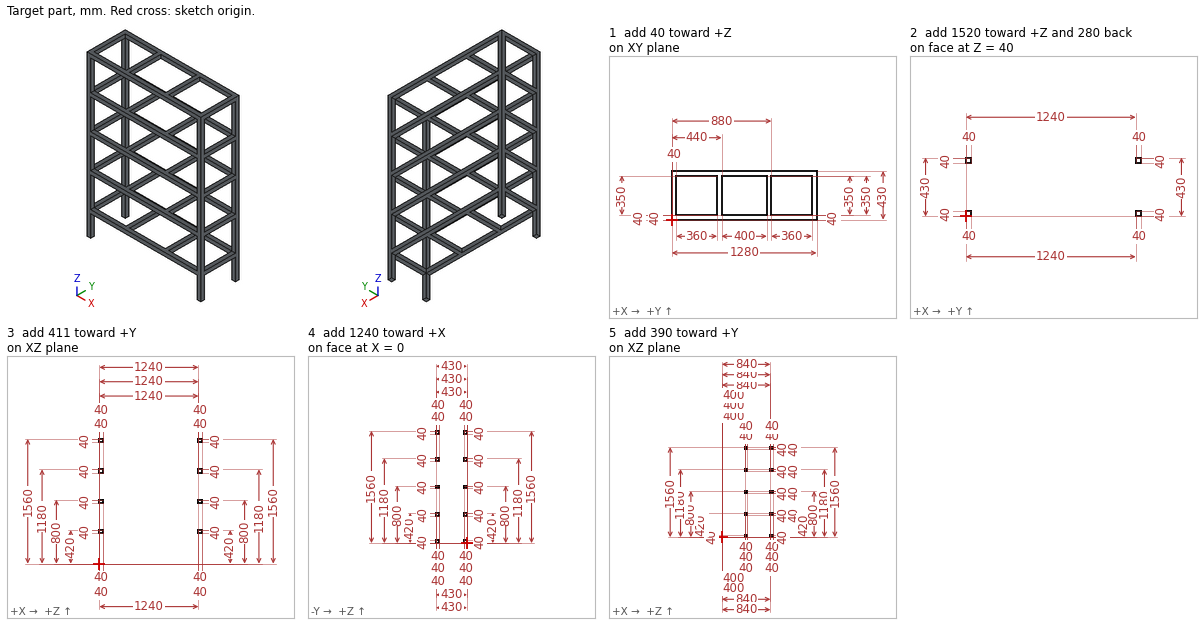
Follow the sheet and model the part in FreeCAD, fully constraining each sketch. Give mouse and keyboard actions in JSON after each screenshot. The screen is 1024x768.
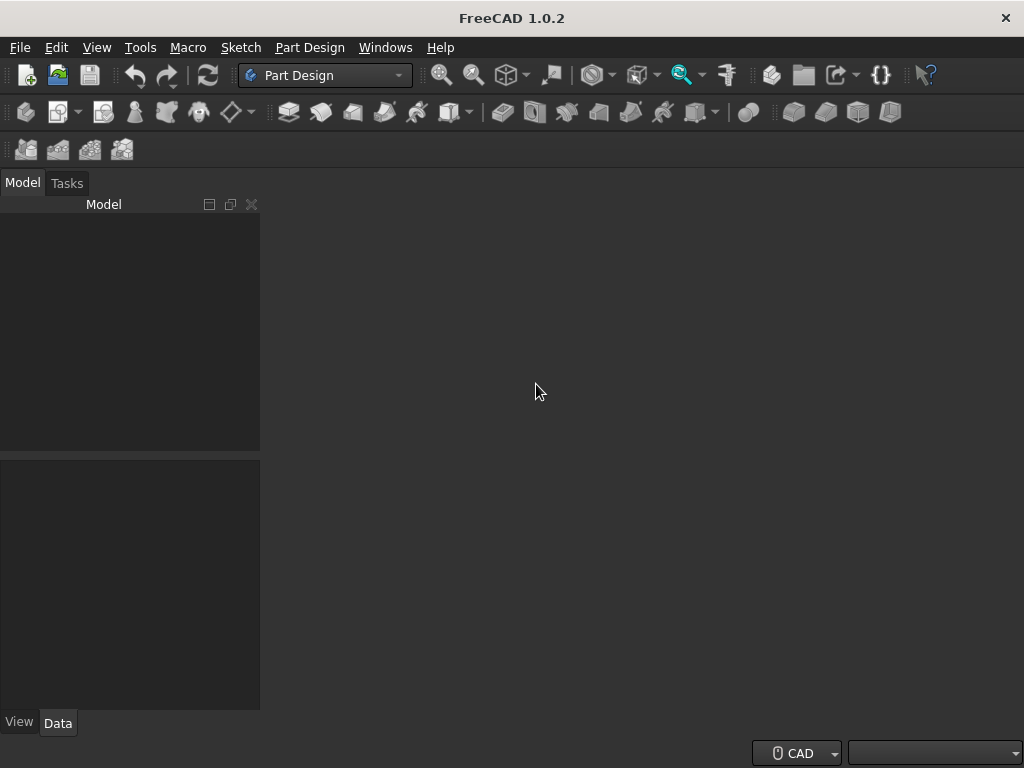
{"action": "left_click", "coordinate": [26, 76]}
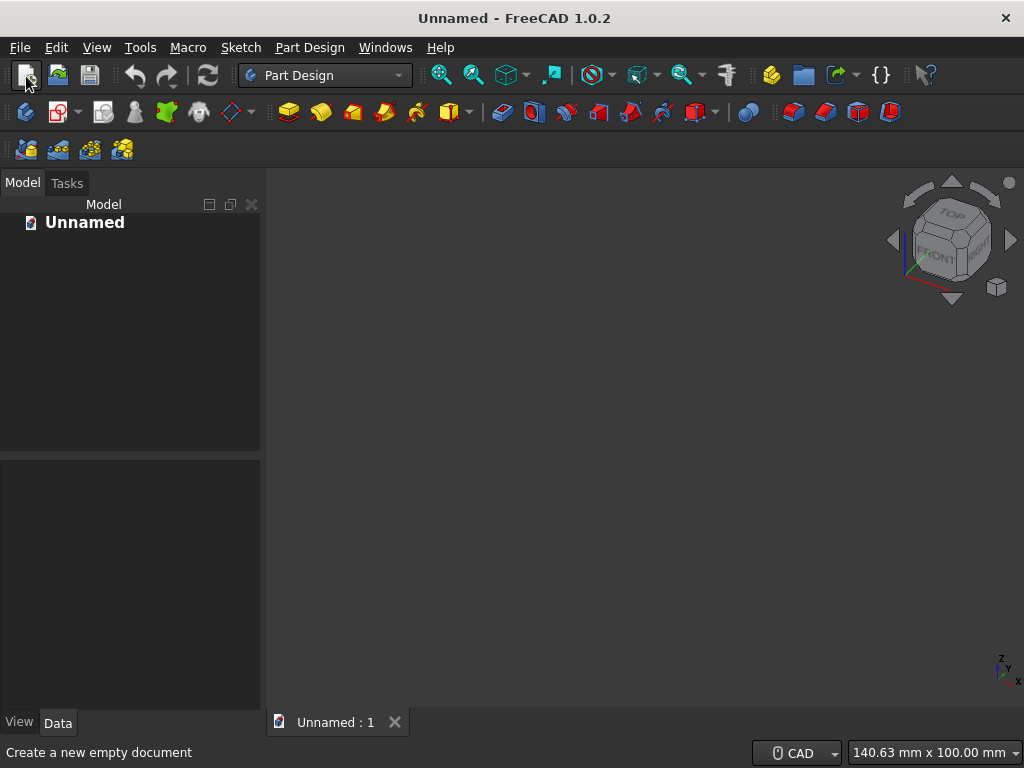
{"action": "left_click", "coordinate": [58, 112]}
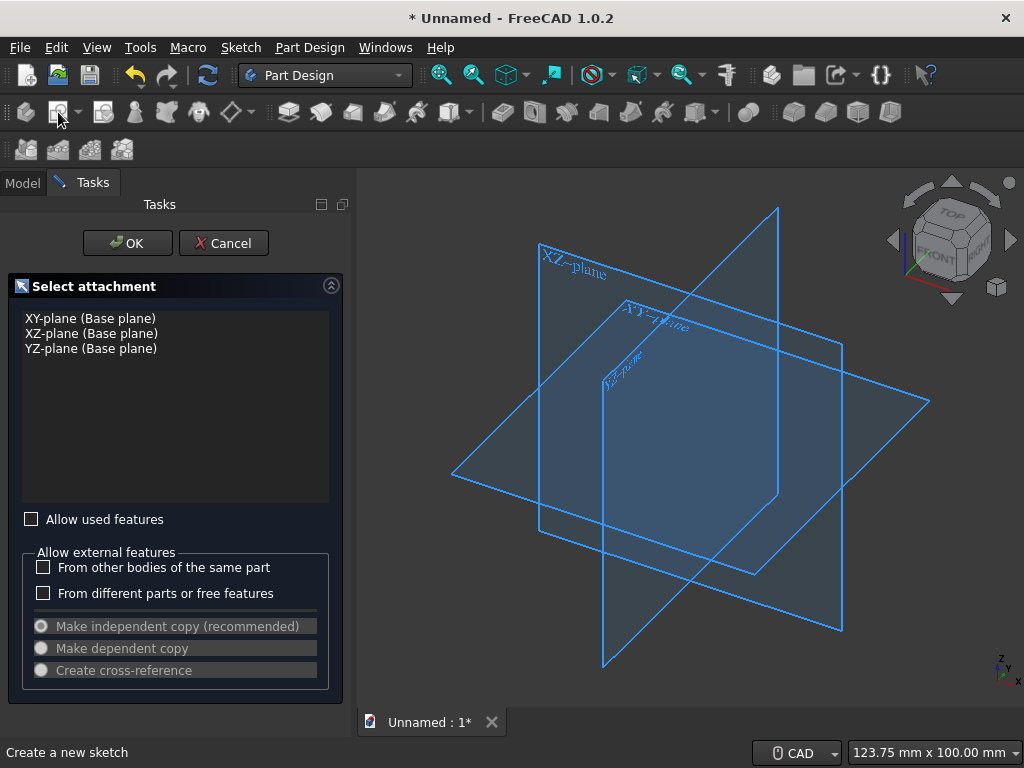
{"action": "left_click", "coordinate": [82, 318]}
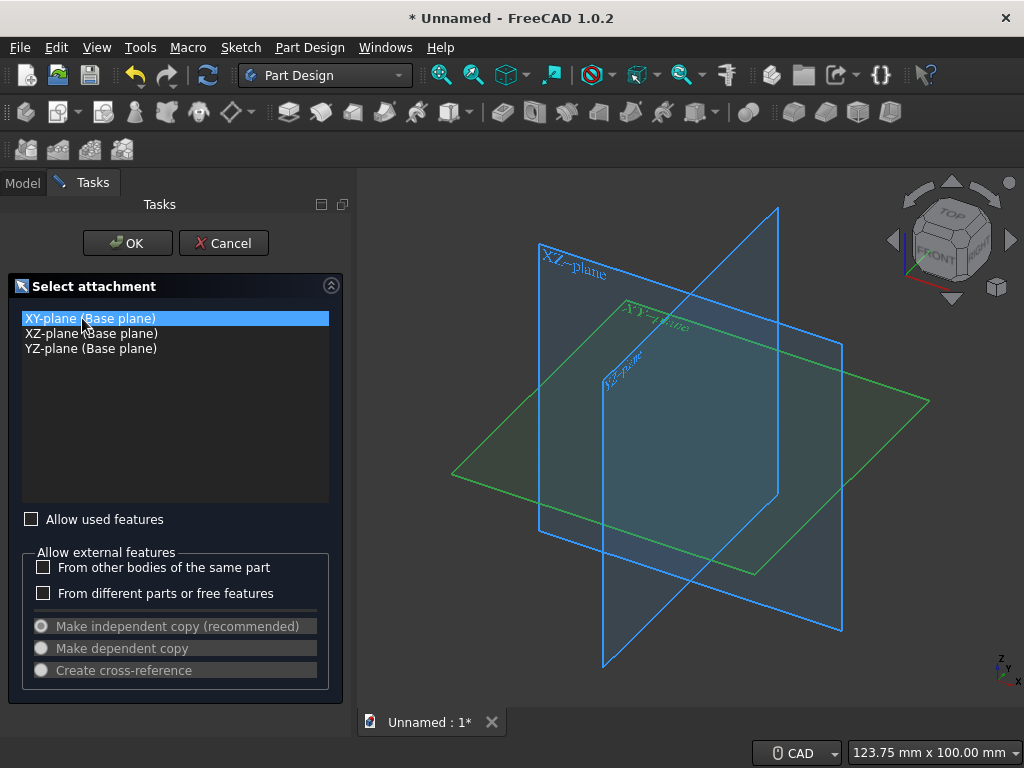
{"action": "left_click", "coordinate": [128, 243]}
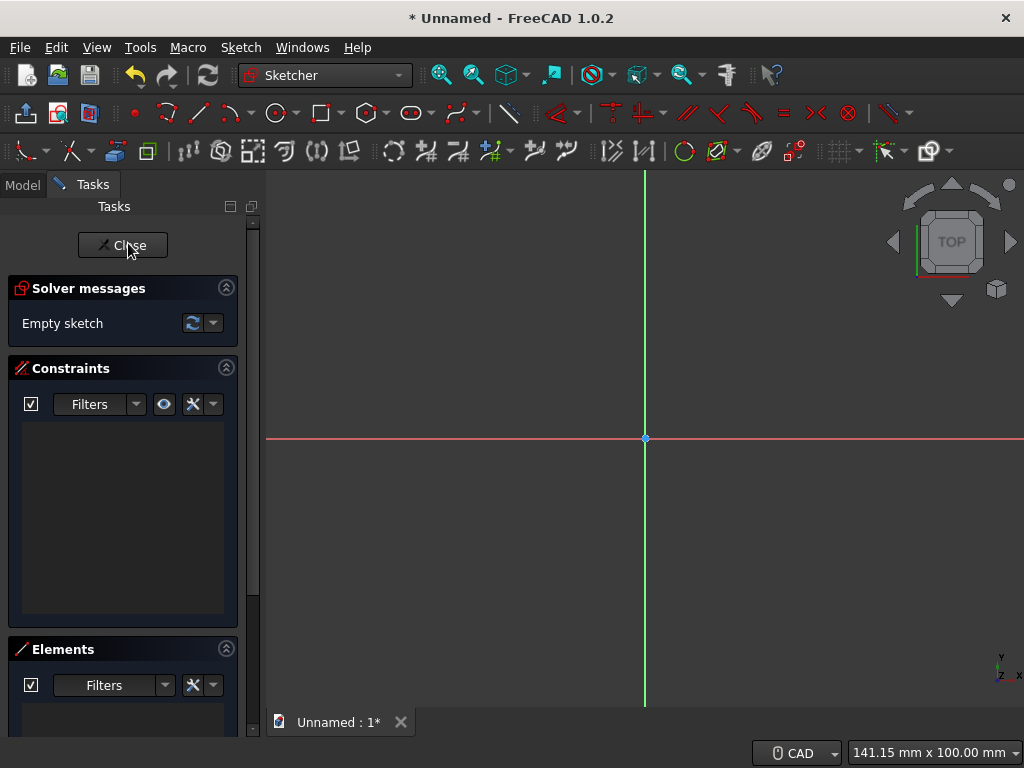
{"action": "scroll", "coordinate": [350, 513], "scroll_direction": "down", "scroll_amount": 14}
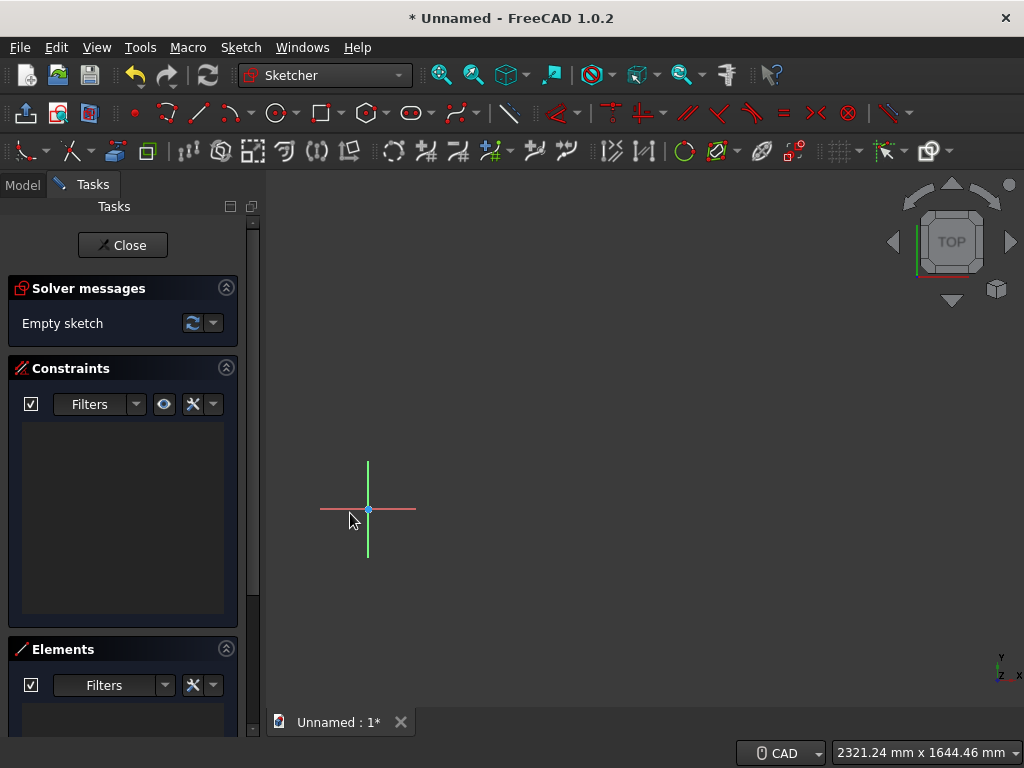
{"action": "left_click", "coordinate": [322, 114]}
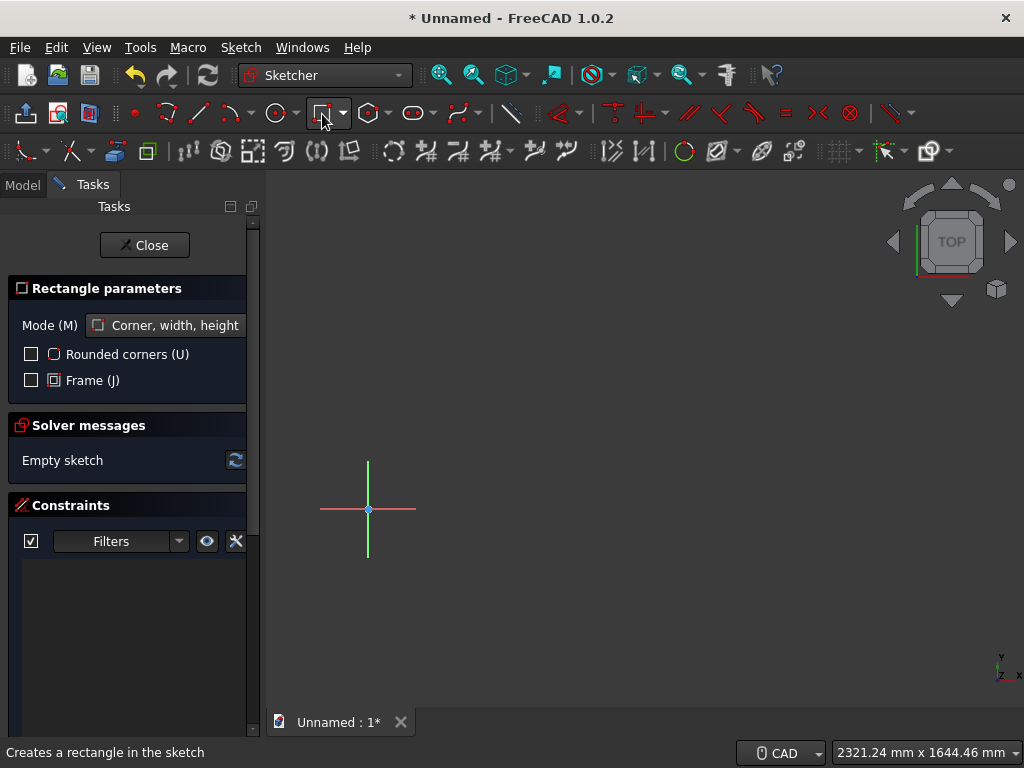
{"action": "left_click", "coordinate": [368, 509]}
{"action": "mouse_move", "coordinate": [786, 369]}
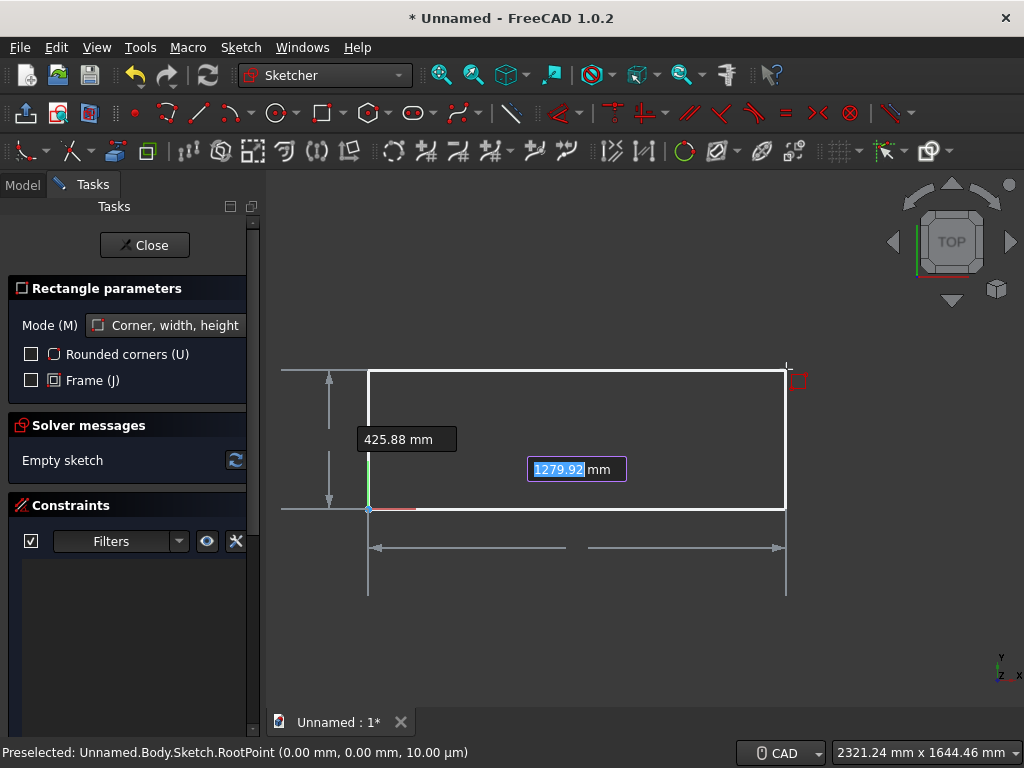
{"action": "type", "text": "1280"}
{"action": "key", "text": "Tab"}
{"action": "type", "text": "430"}
{"action": "key", "text": "Return"}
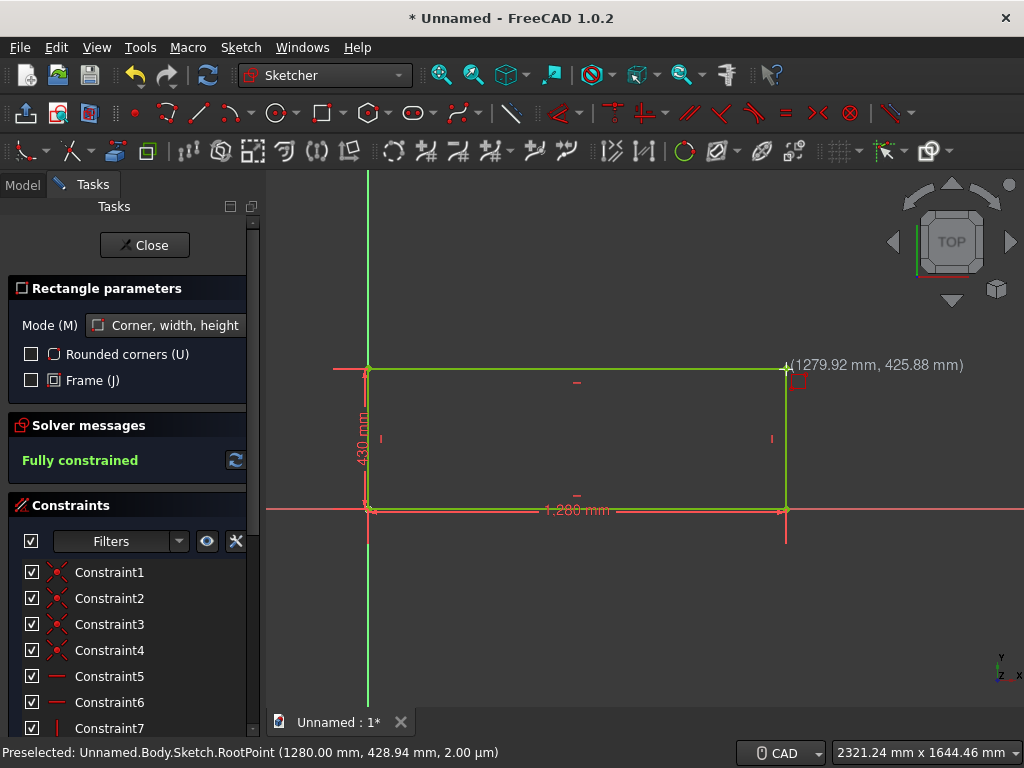
{"action": "left_click", "coordinate": [381, 382]}
{"action": "mouse_move", "coordinate": [499, 496]}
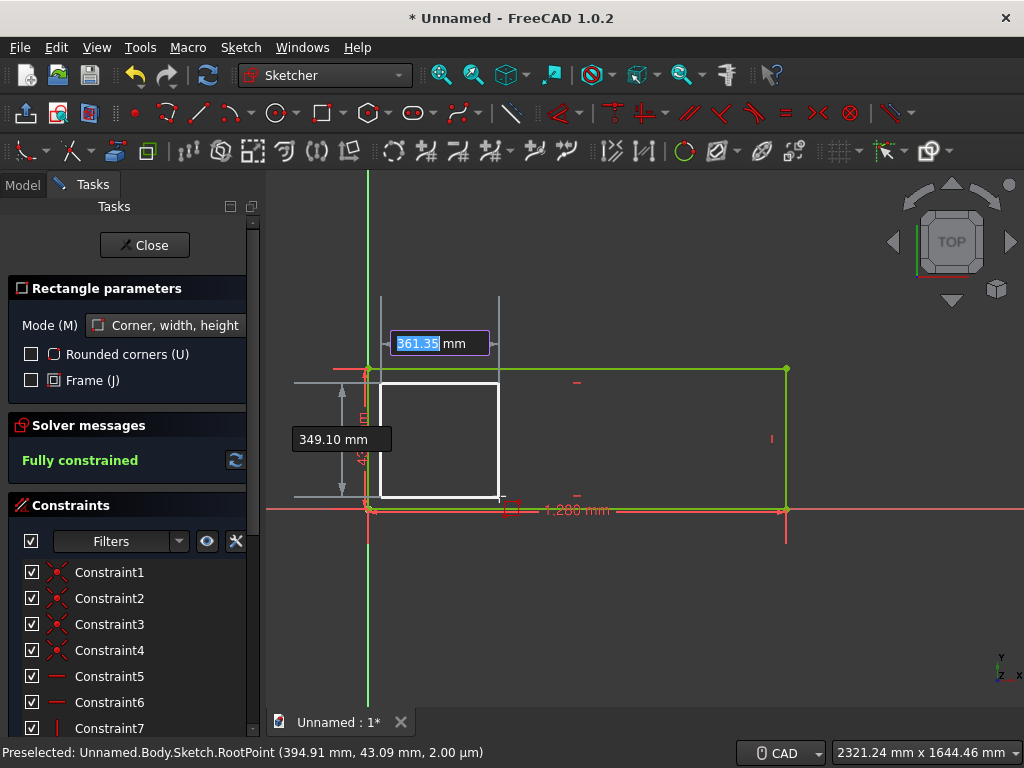
{"action": "type", "text": "360"}
{"action": "key", "text": "Tab"}
{"action": "type", "text": "350"}
{"action": "key", "text": "Return"}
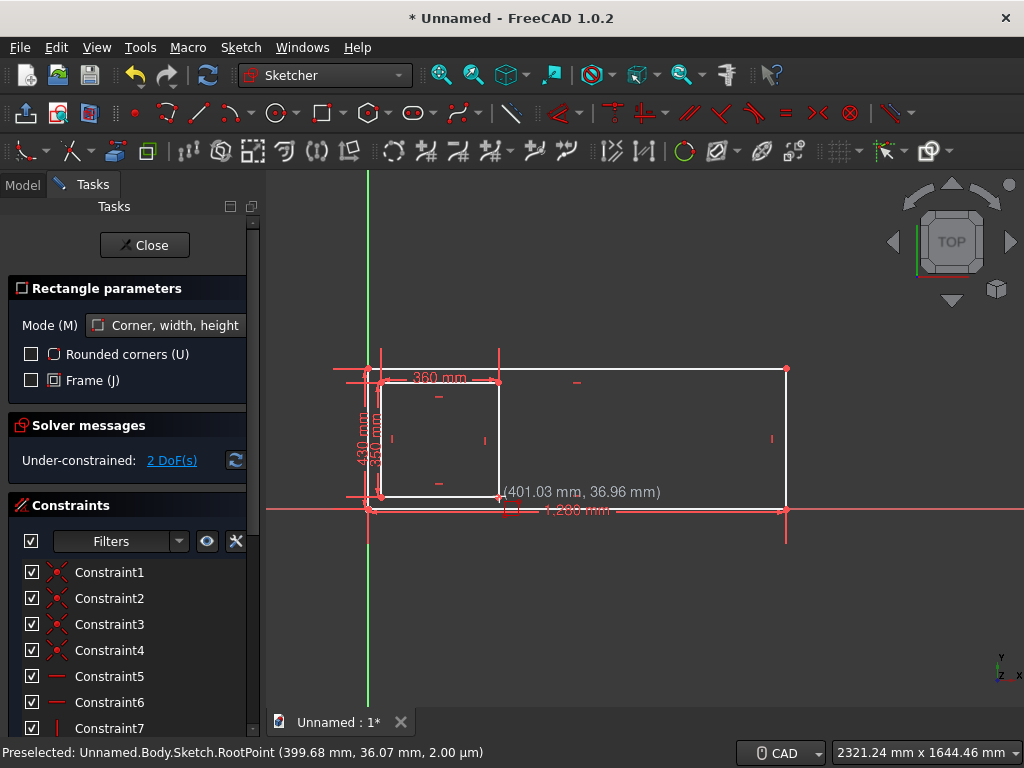
{"action": "left_click", "coordinate": [512, 382]}
{"action": "mouse_move", "coordinate": [642, 496]}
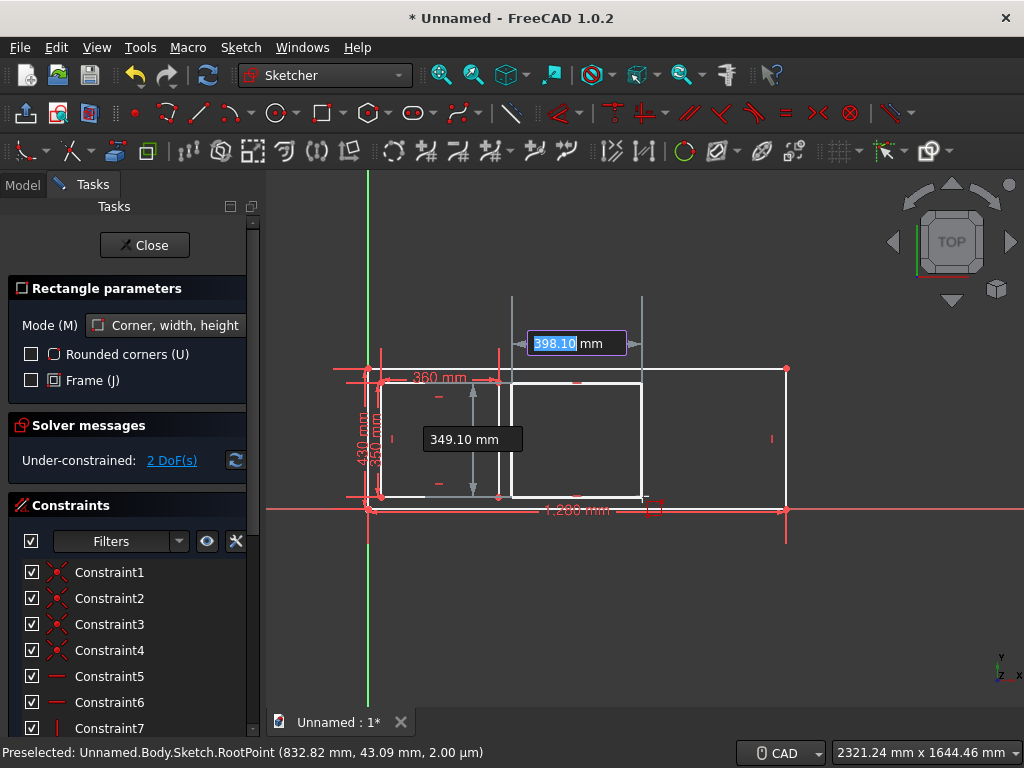
{"action": "type", "text": "400"}
{"action": "key", "text": "Tab"}
{"action": "type", "text": "350"}
{"action": "key", "text": "Return"}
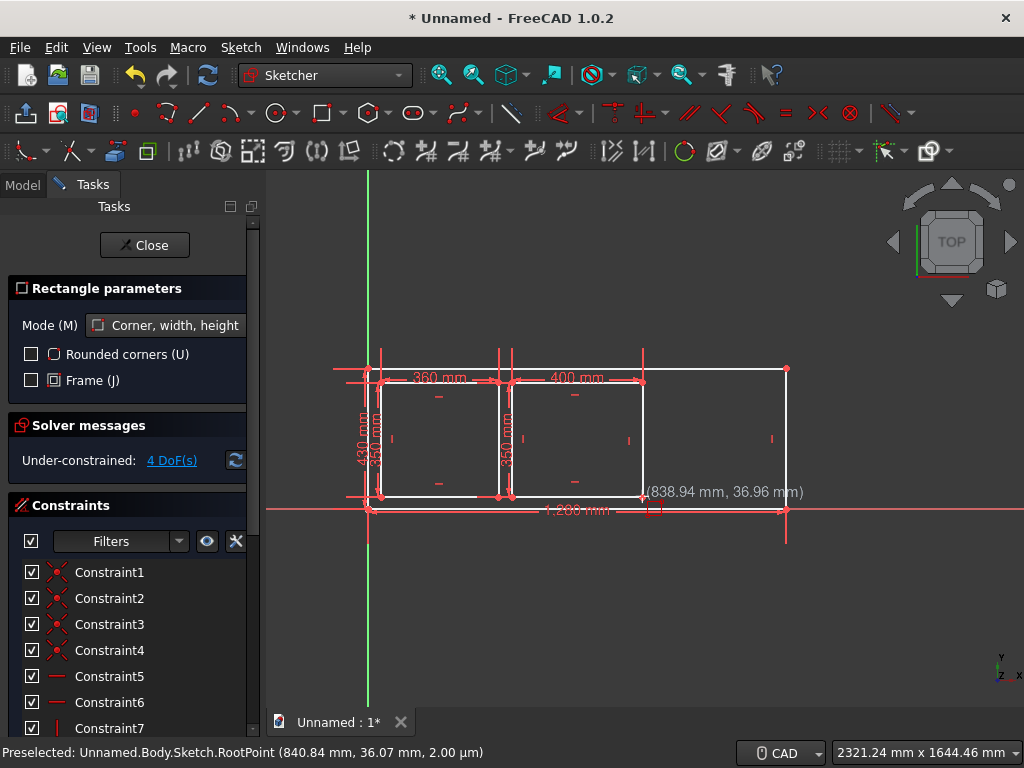
{"action": "left_click", "coordinate": [655, 382]}
{"action": "mouse_move", "coordinate": [773, 496]}